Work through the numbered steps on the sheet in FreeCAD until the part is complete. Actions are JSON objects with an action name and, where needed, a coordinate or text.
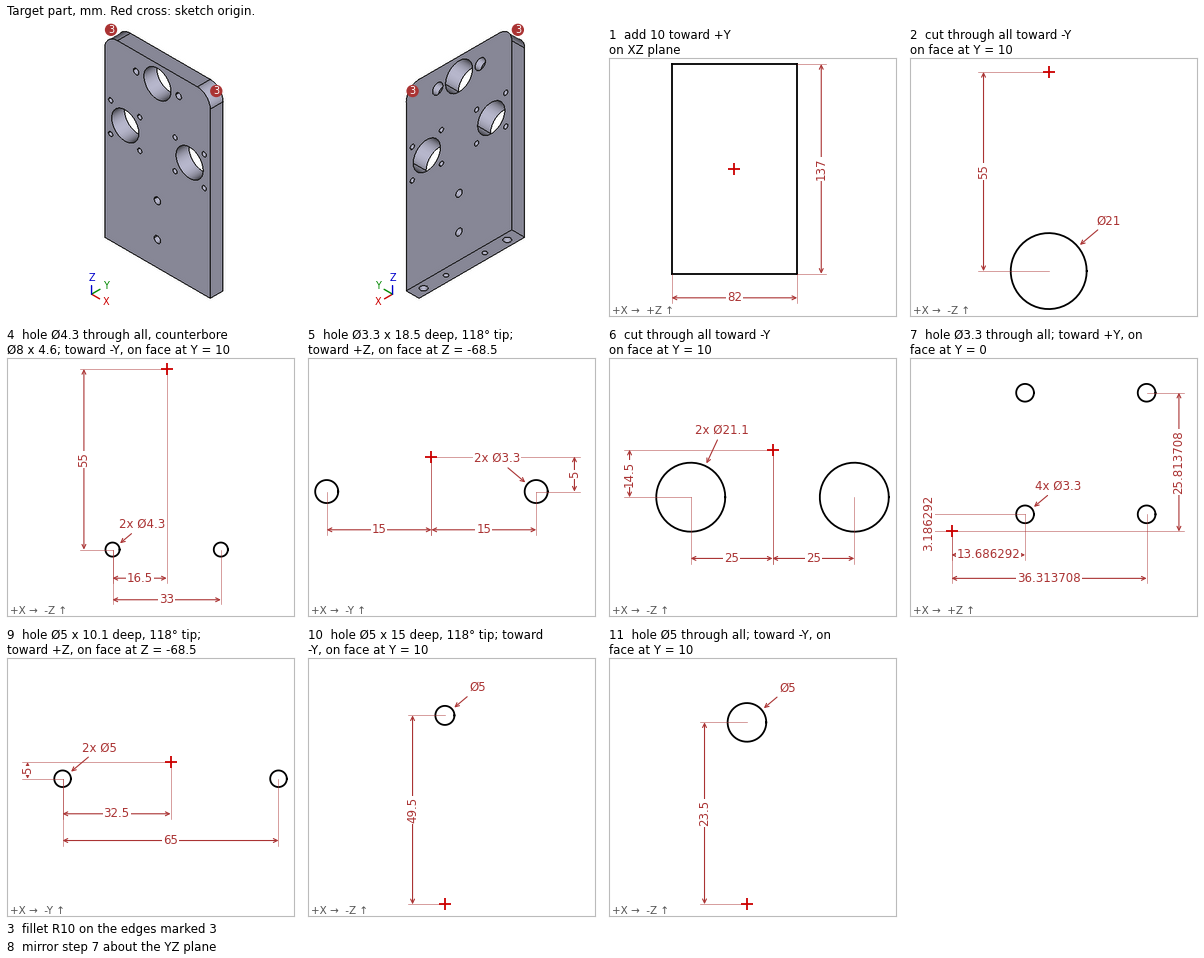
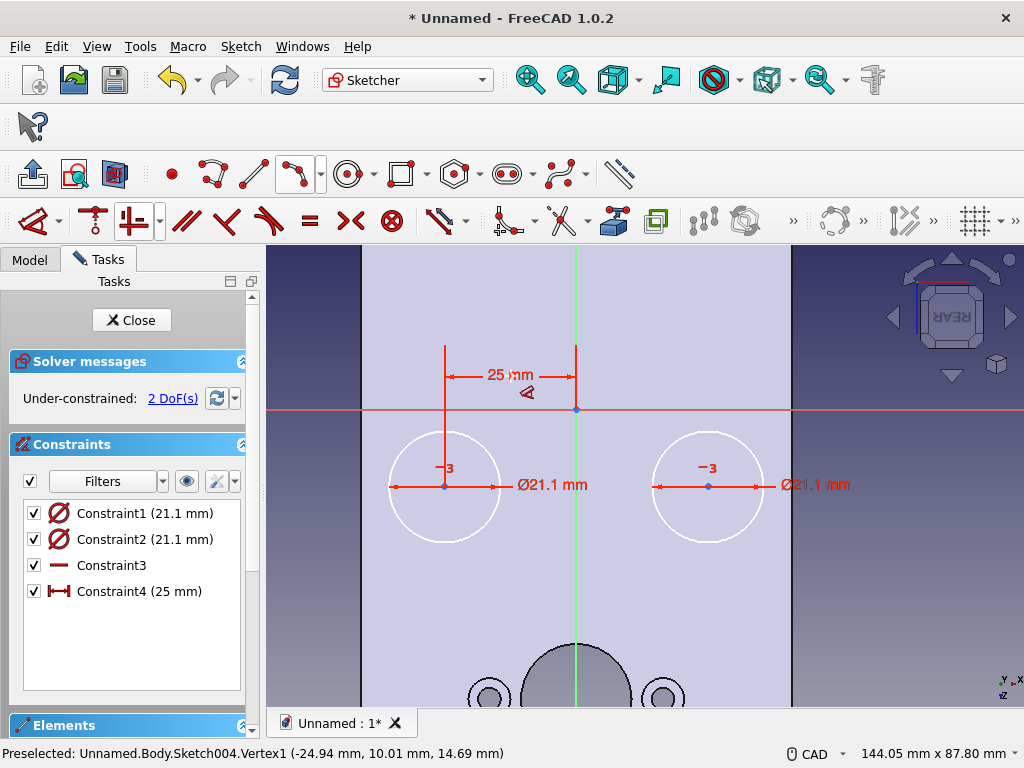
{"action": "left_click", "coordinate": [708, 487]}
{"action": "left_click", "coordinate": [642, 376]}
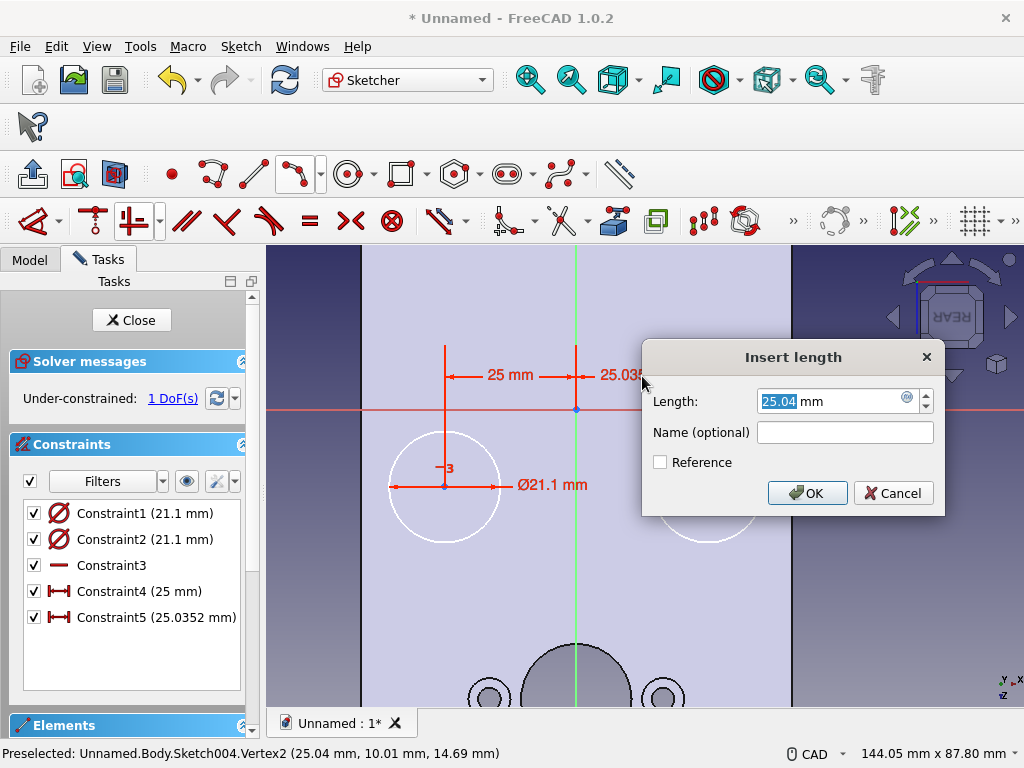
{"action": "type", "text": "25"}
{"action": "key", "text": "Return"}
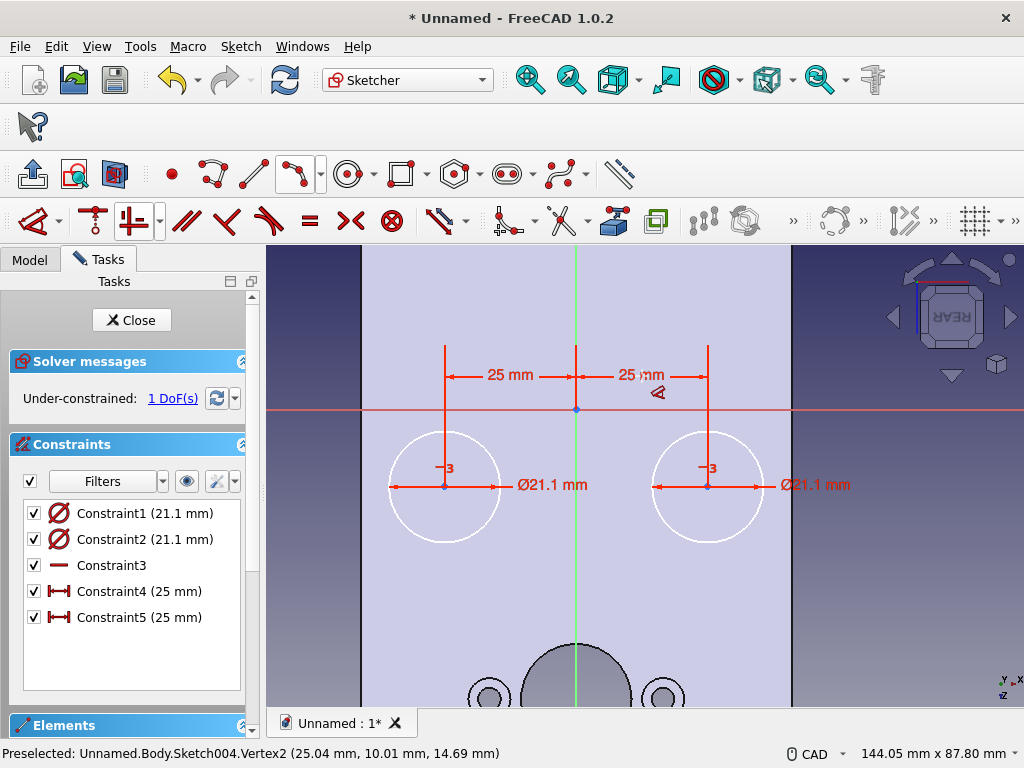
{"action": "left_click", "coordinate": [445, 487]}
{"action": "left_click", "coordinate": [411, 466]}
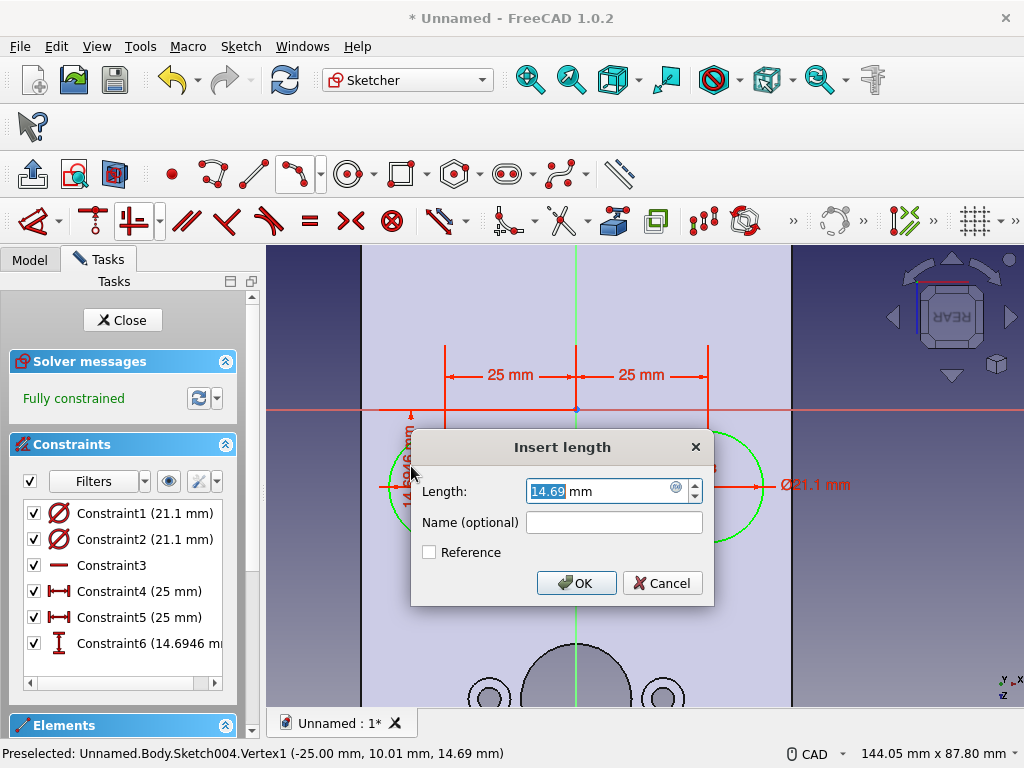
{"action": "type", "text": "14.5"}
{"action": "key", "text": "Return"}
{"action": "key", "text": "Escape"}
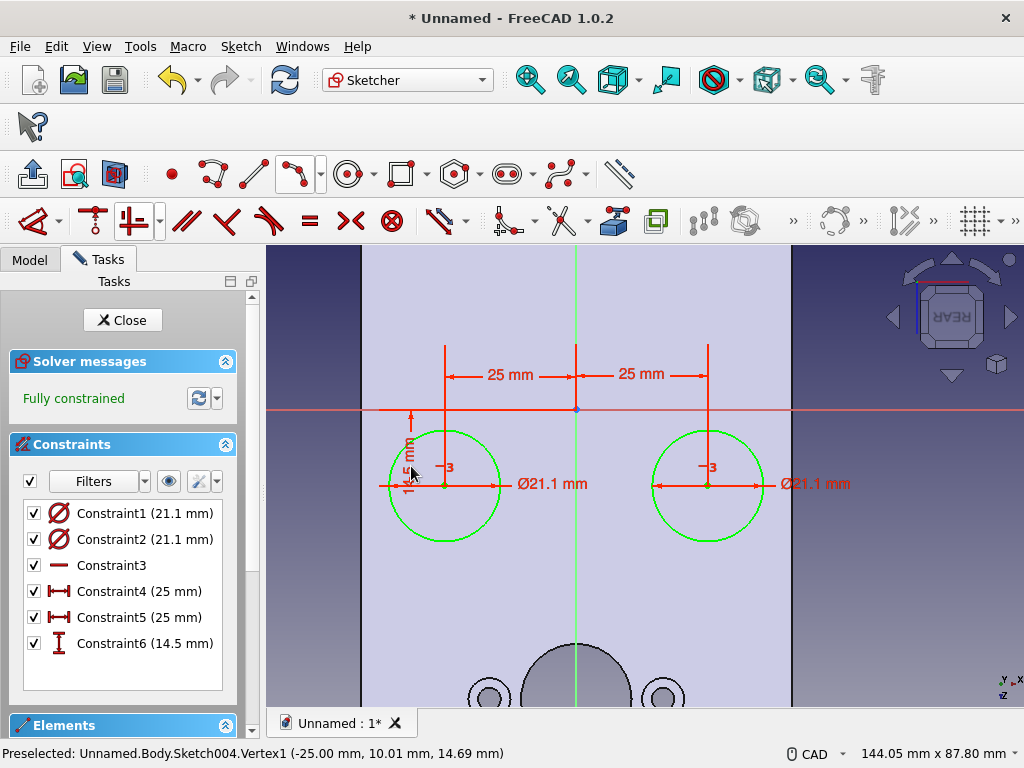
{"action": "left_click", "coordinate": [123, 320]}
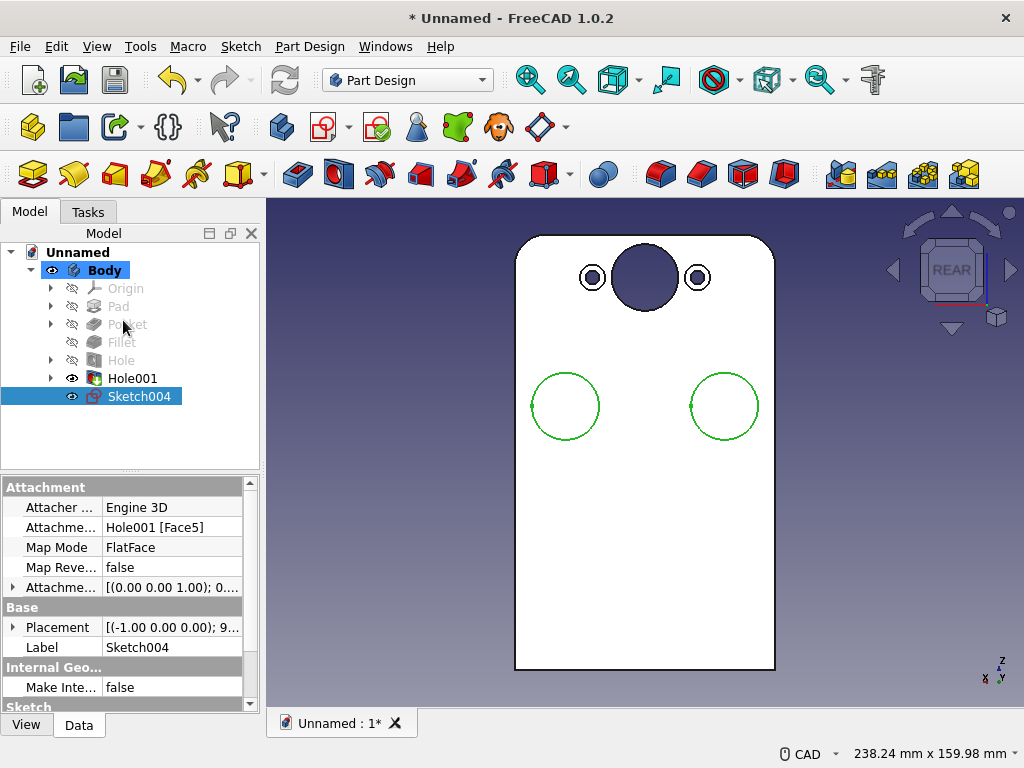
{"action": "left_click", "coordinate": [298, 174]}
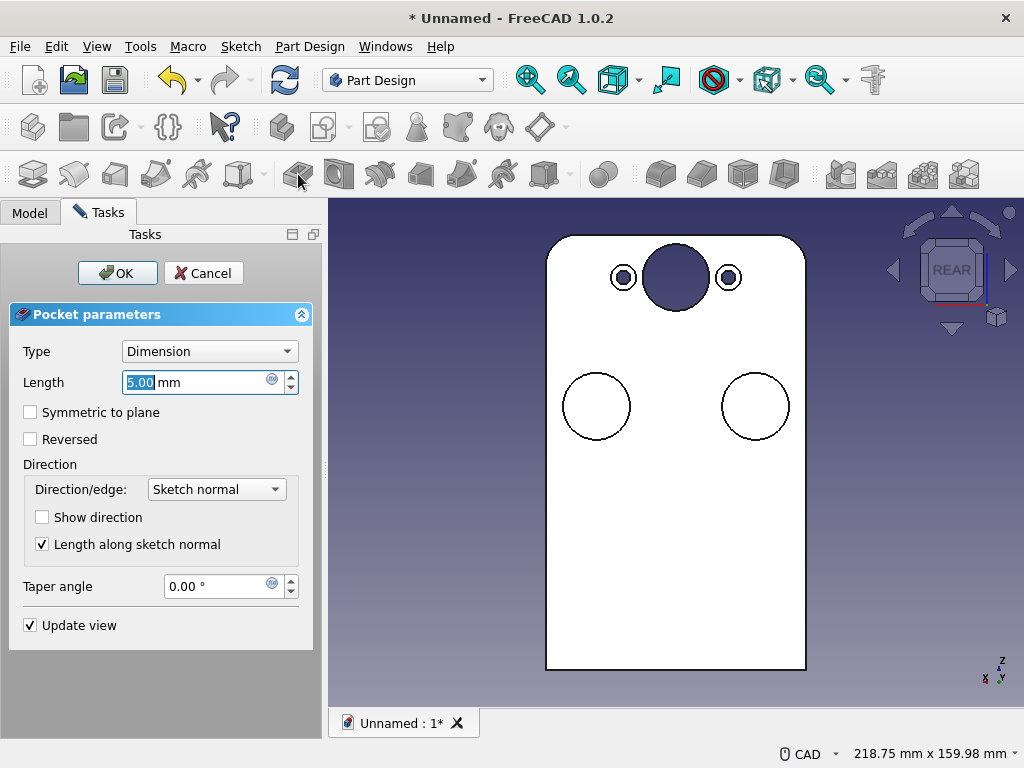
{"action": "left_click", "coordinate": [210, 352]}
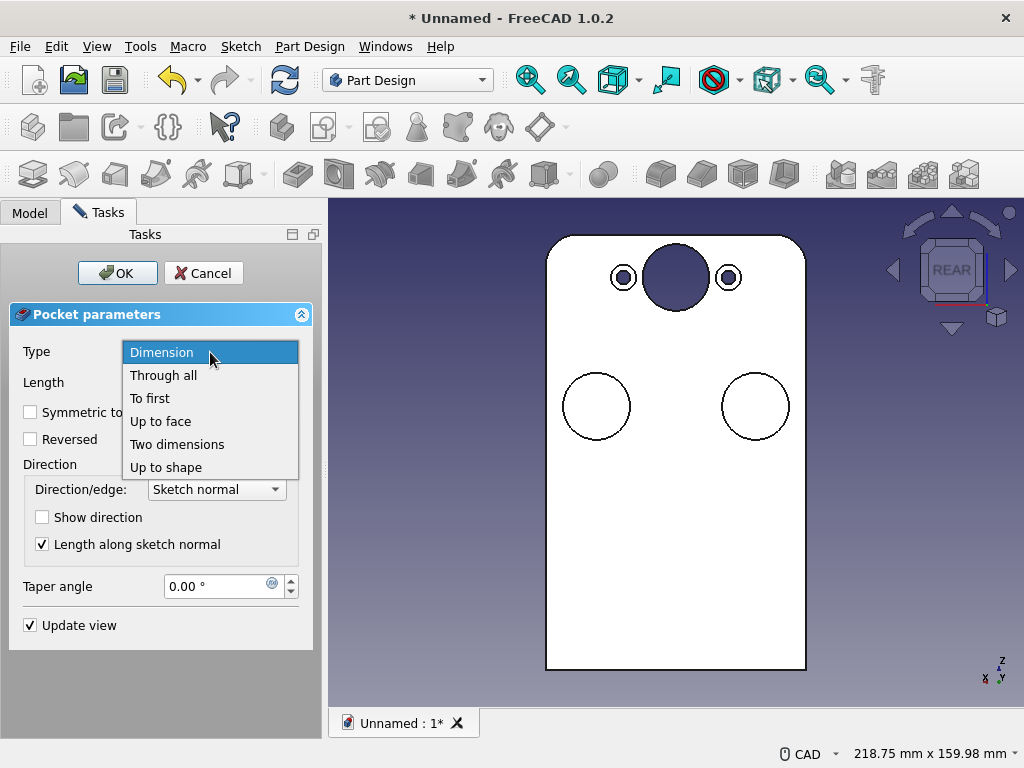
{"action": "left_click", "coordinate": [208, 376]}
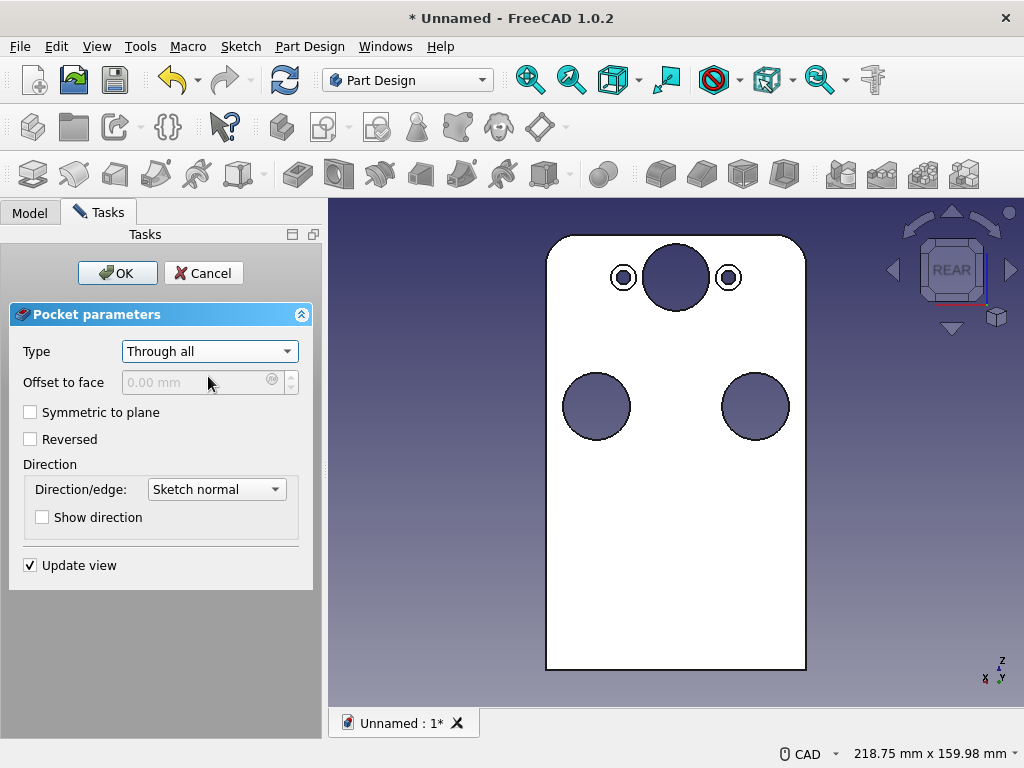
{"action": "left_click", "coordinate": [118, 273]}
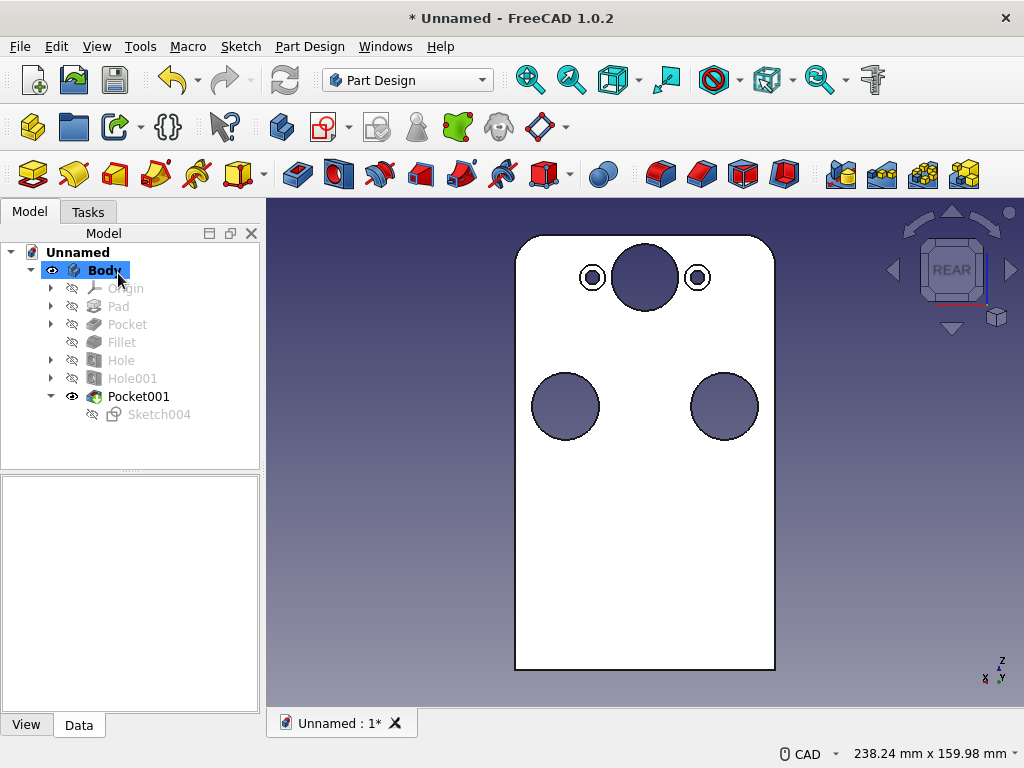
{"action": "key", "text": "0"}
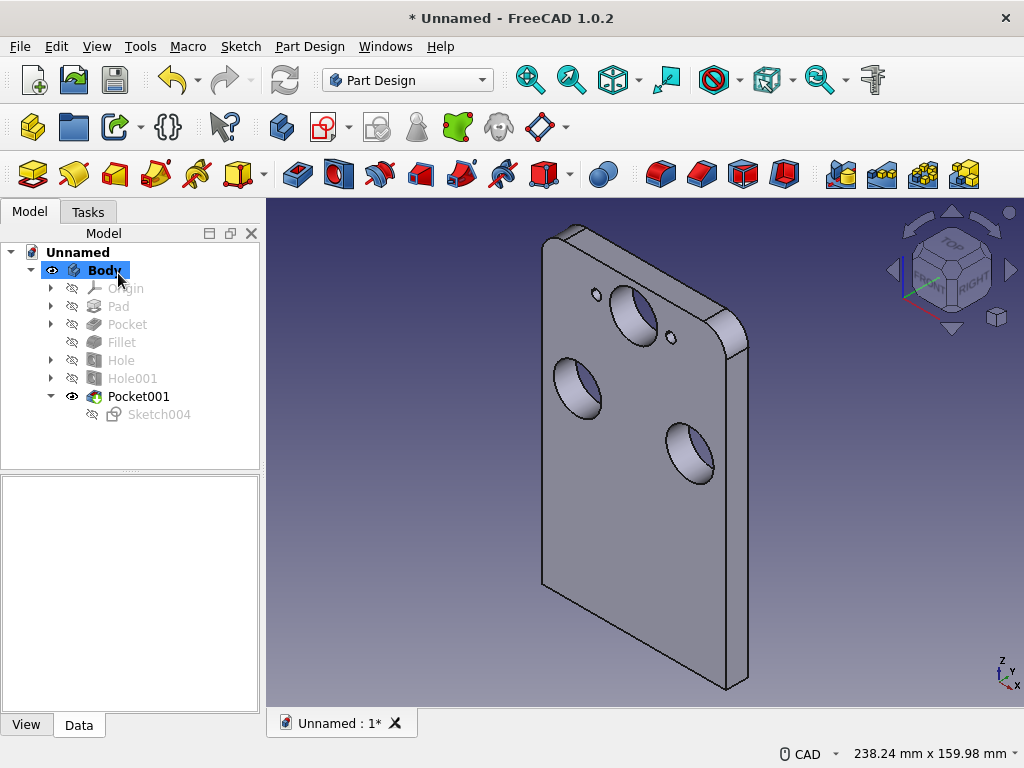
{"action": "left_click", "coordinate": [634, 509]}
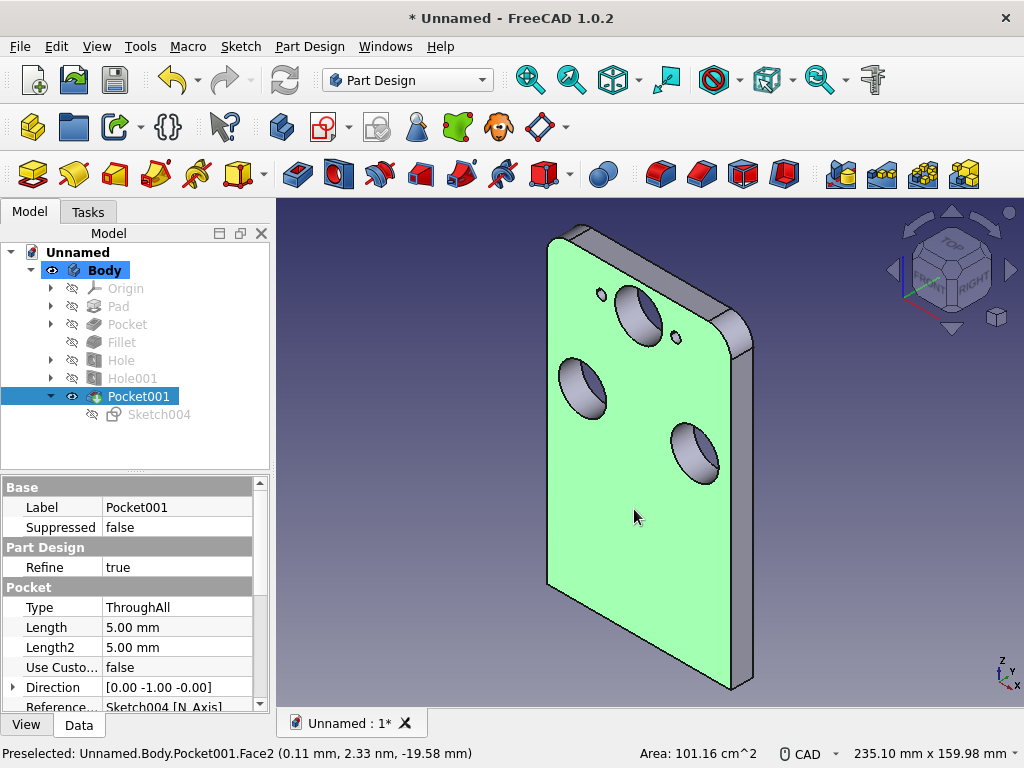
{"action": "left_click", "coordinate": [322, 128]}